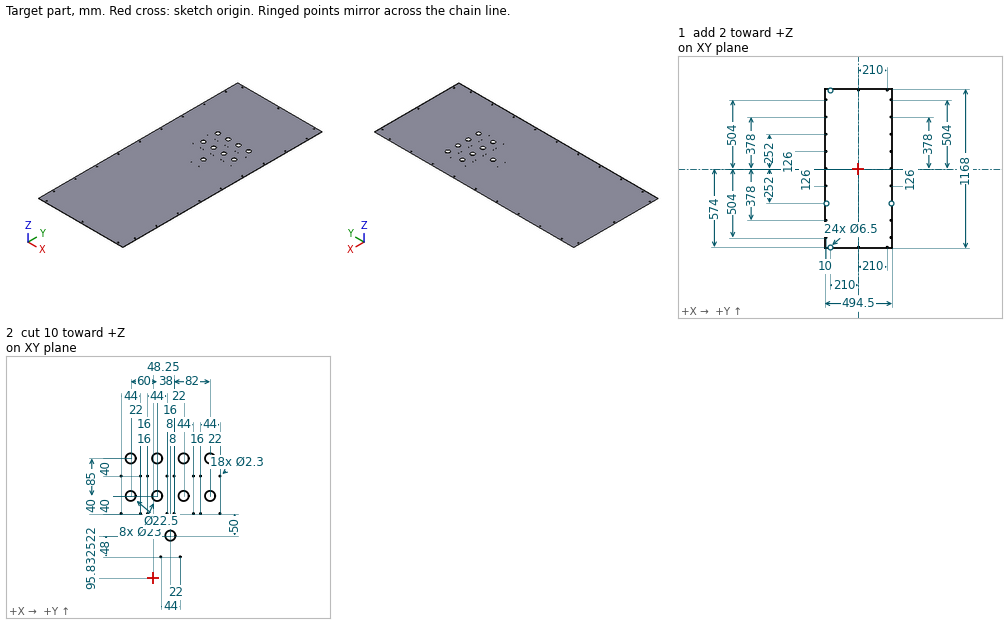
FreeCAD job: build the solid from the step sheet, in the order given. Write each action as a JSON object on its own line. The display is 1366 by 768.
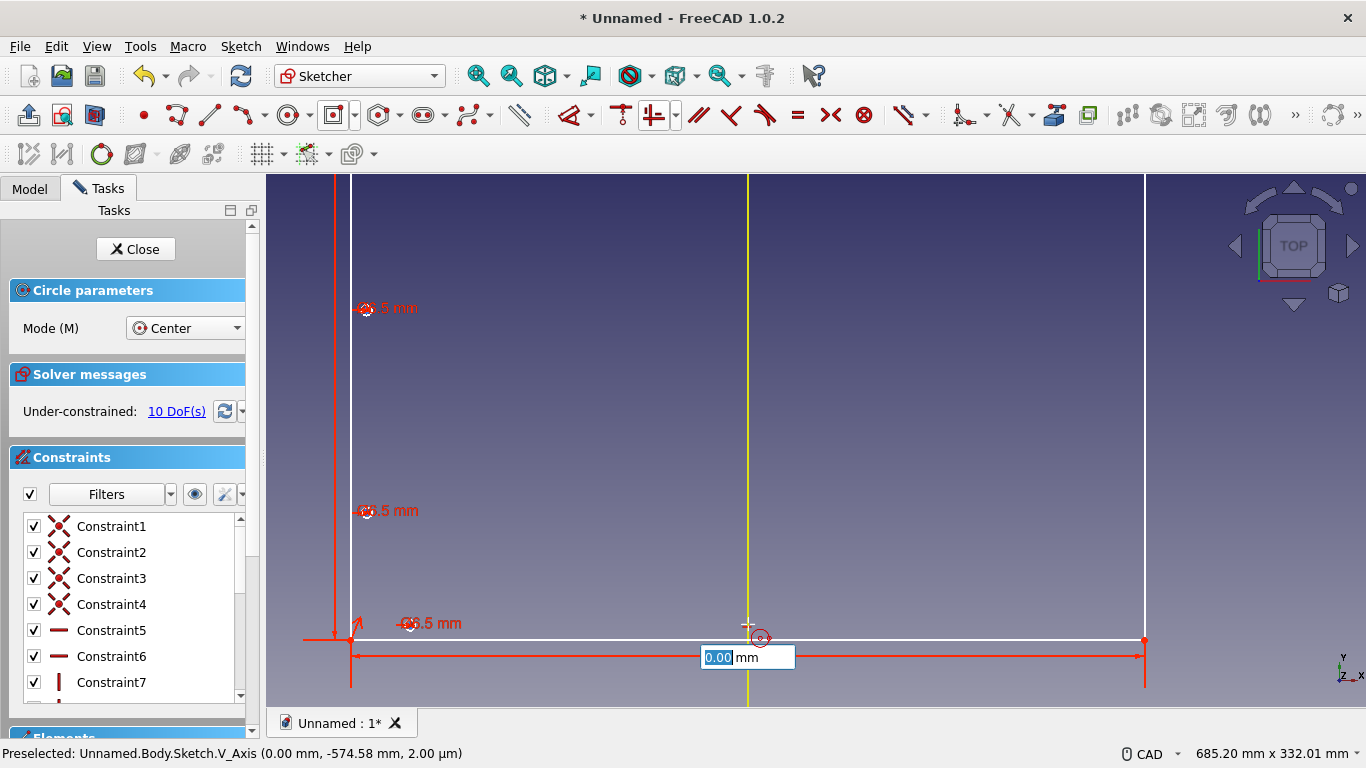
{"action": "scroll", "coordinate": [753, 622], "scroll_direction": "up", "scroll_amount": 6}
{"action": "mouse_move", "coordinate": [750, 621]}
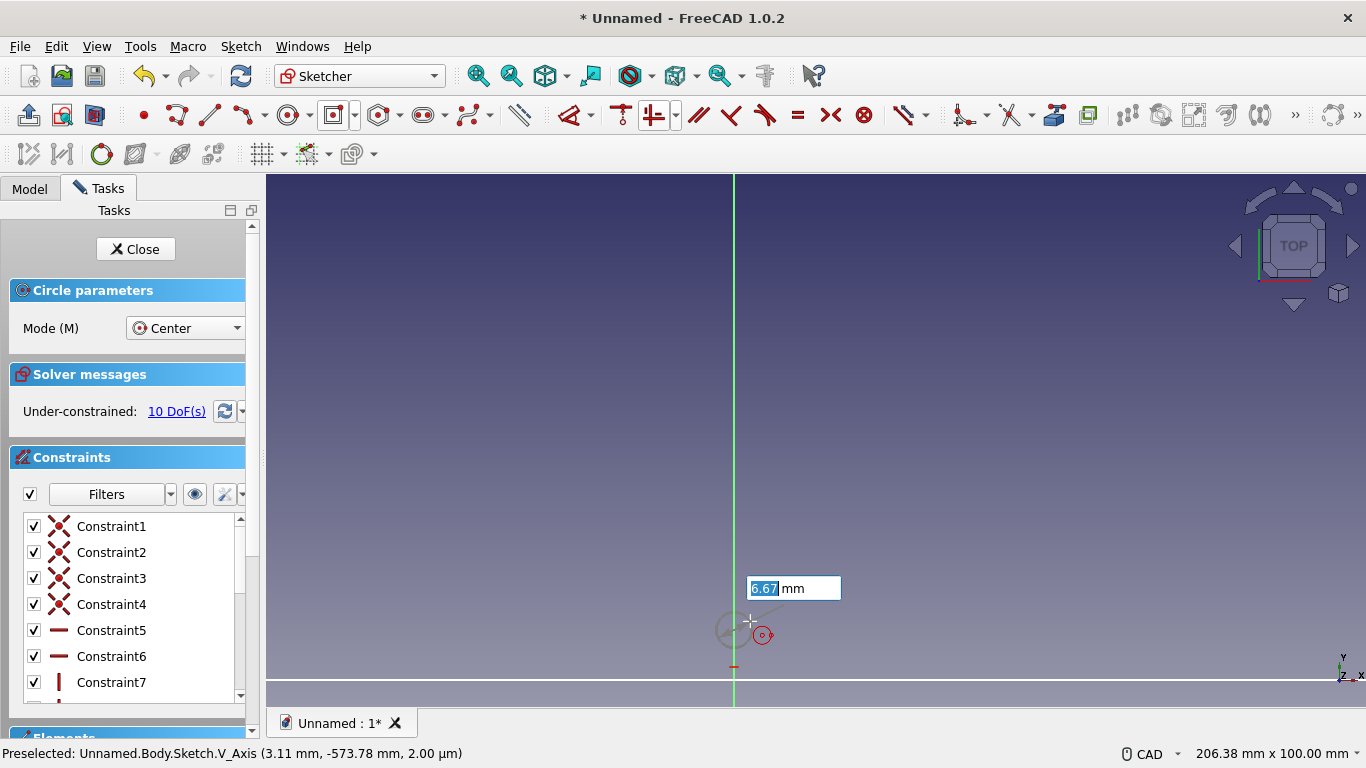
{"action": "type", "text": "6.5"}
{"action": "key", "text": "Return"}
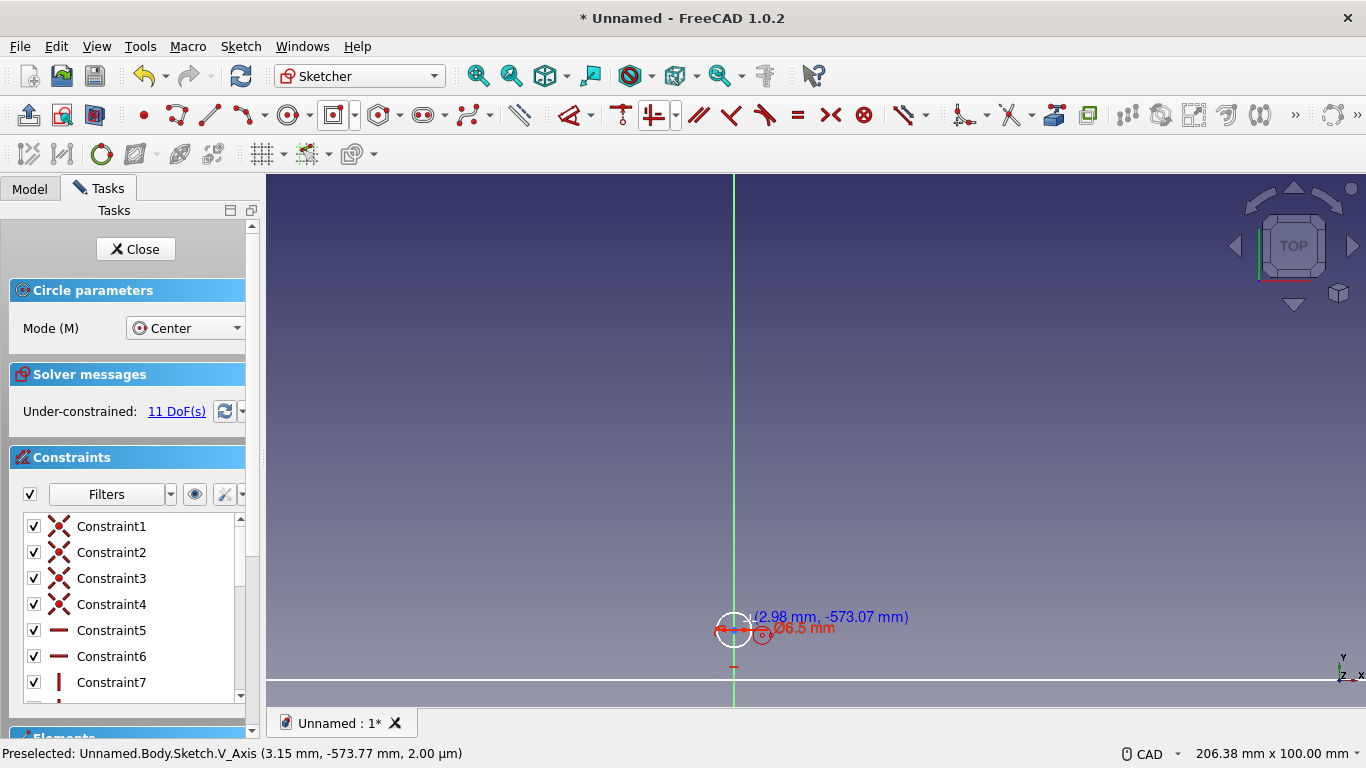
{"action": "scroll", "coordinate": [748, 591], "scroll_direction": "down", "scroll_amount": 15}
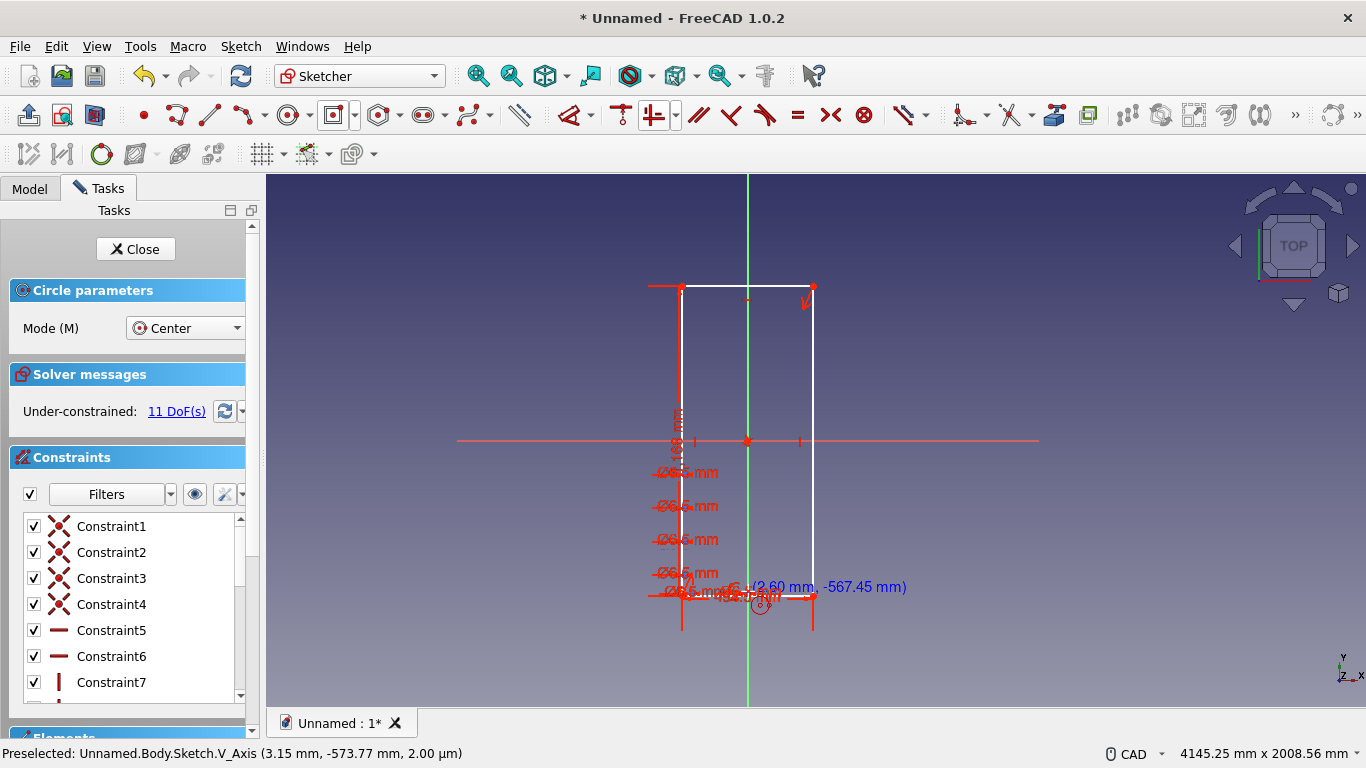
{"action": "scroll", "coordinate": [803, 594], "scroll_direction": "up", "scroll_amount": 17}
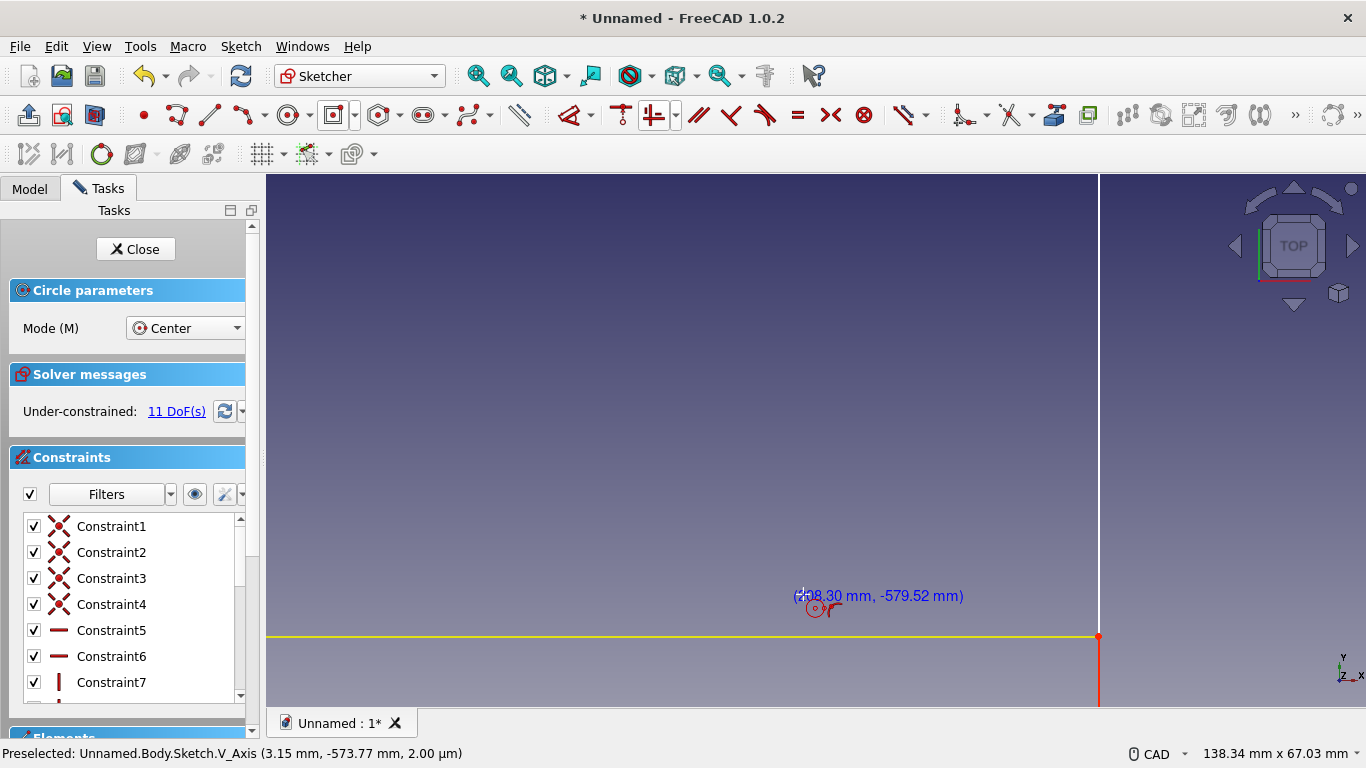
{"action": "scroll", "coordinate": [816, 629], "scroll_direction": "down", "scroll_amount": 16}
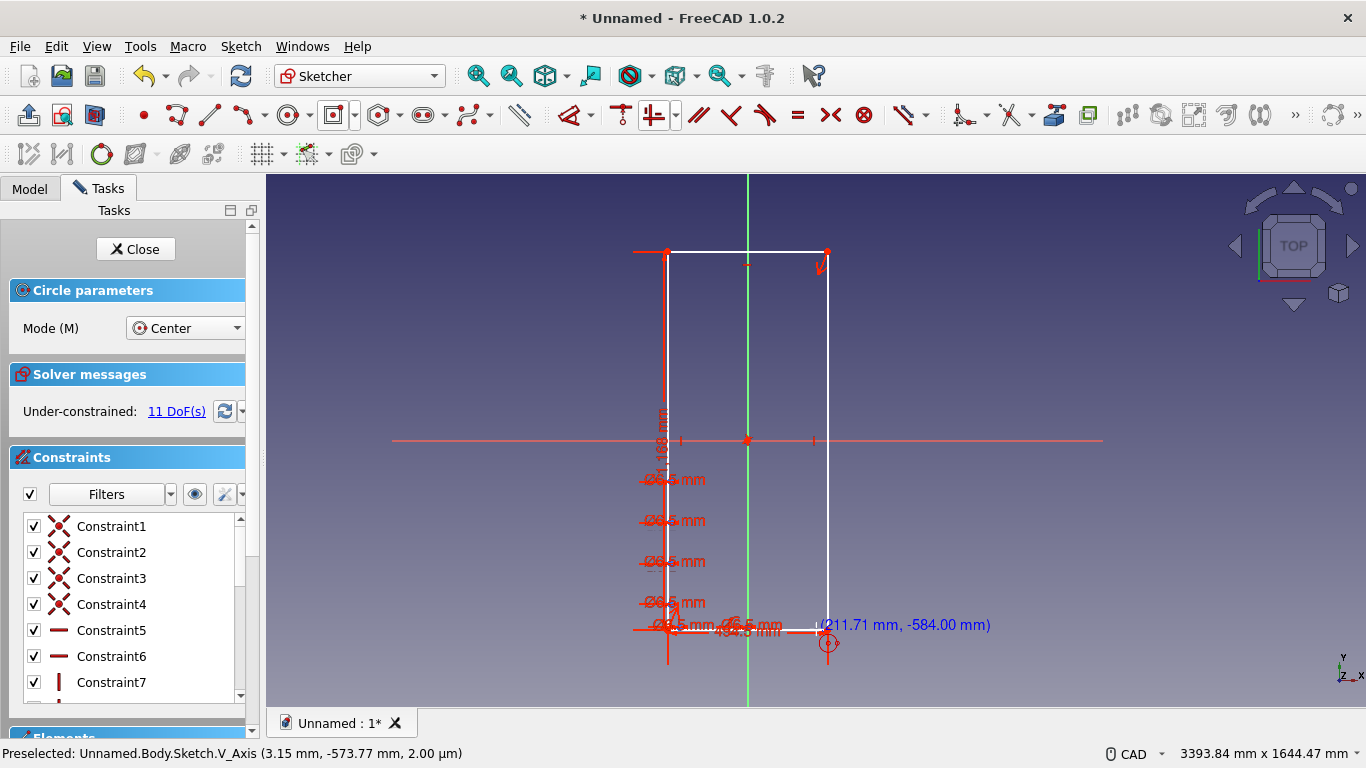
{"action": "scroll", "coordinate": [816, 627], "scroll_direction": "up", "scroll_amount": 8}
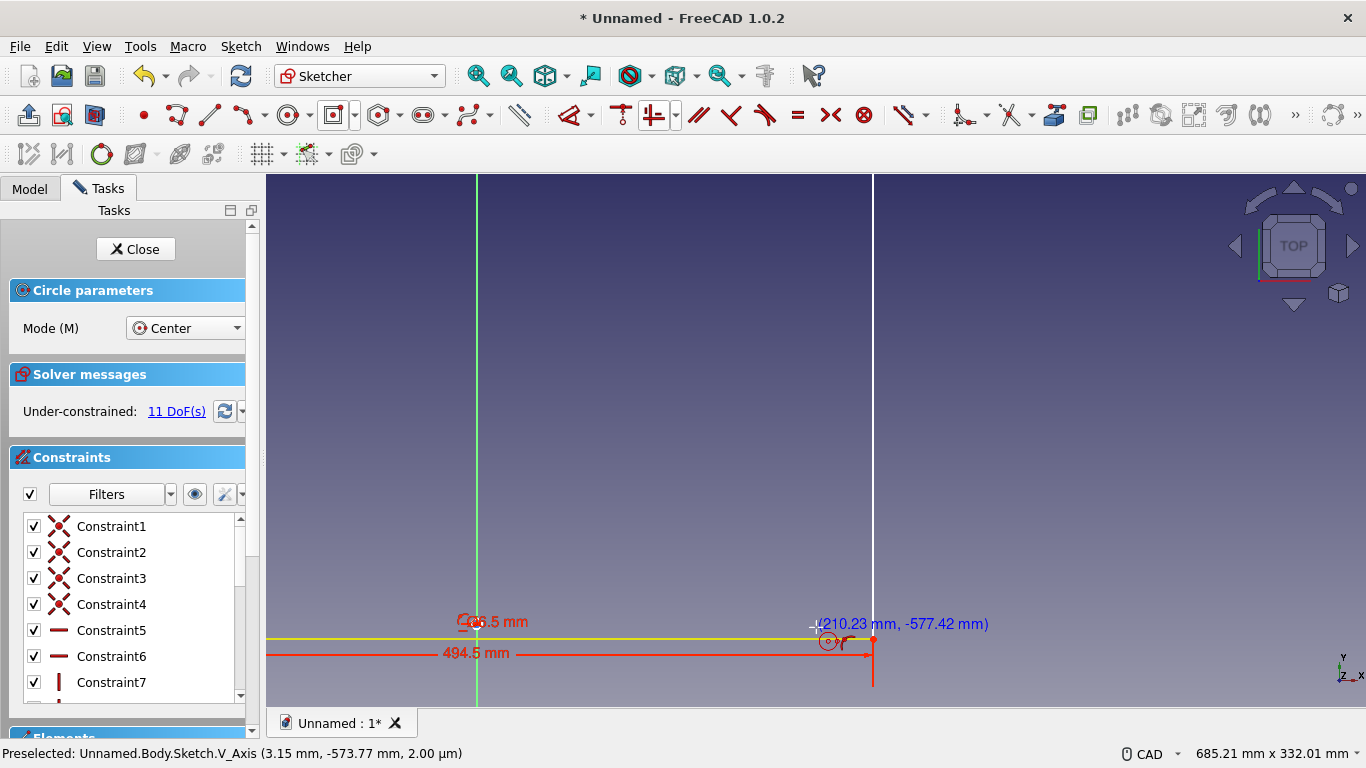
{"action": "left_click", "coordinate": [814, 623]}
{"action": "mouse_move", "coordinate": [817, 619]}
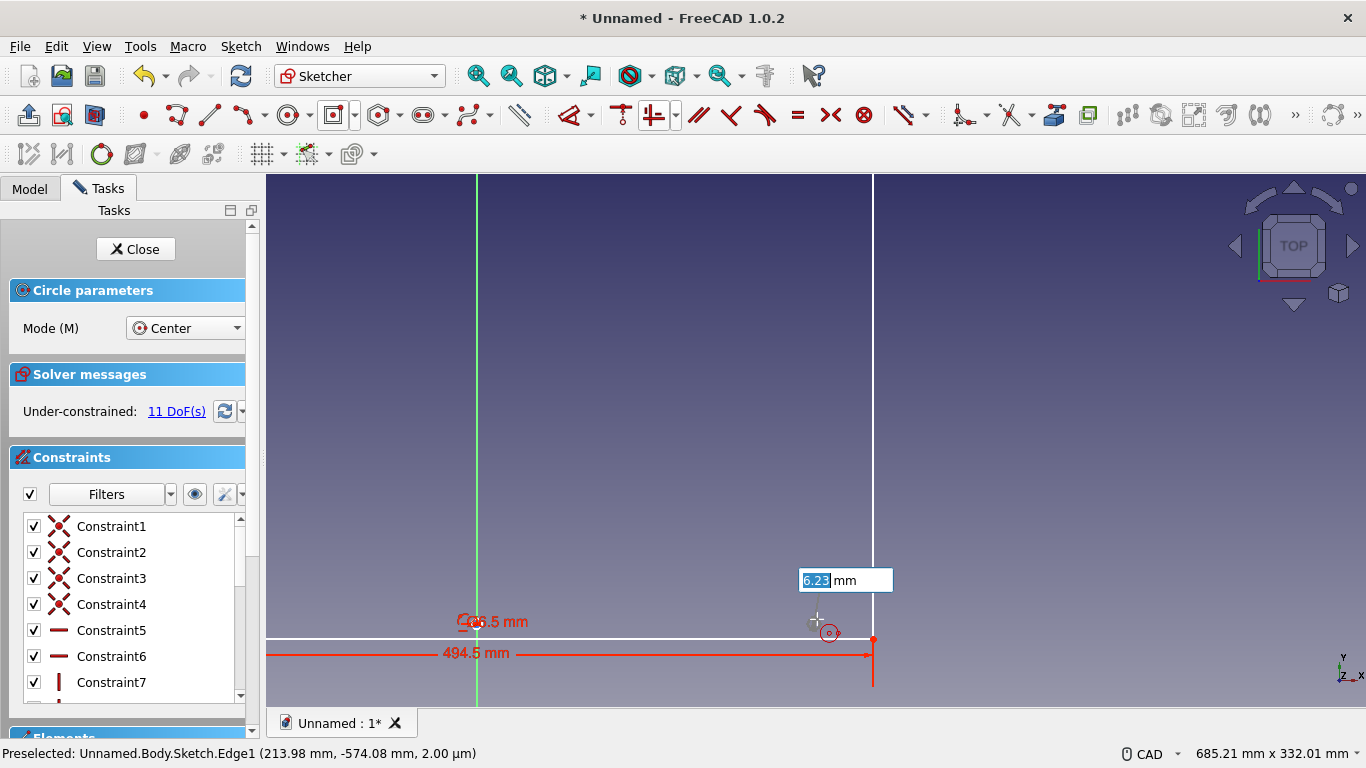
{"action": "type", "text": "6.5"}
{"action": "key", "text": "Return"}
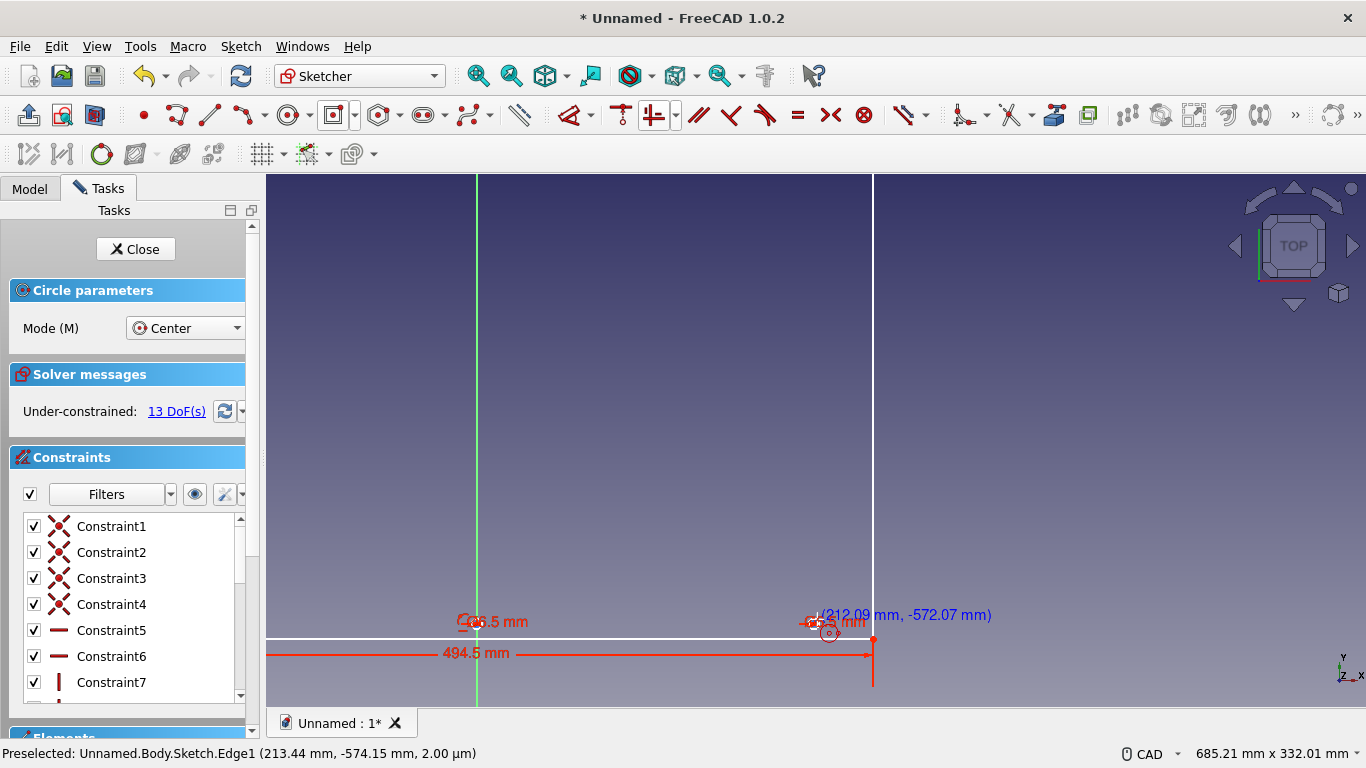
{"action": "scroll", "coordinate": [857, 511], "scroll_direction": "up", "scroll_amount": 8}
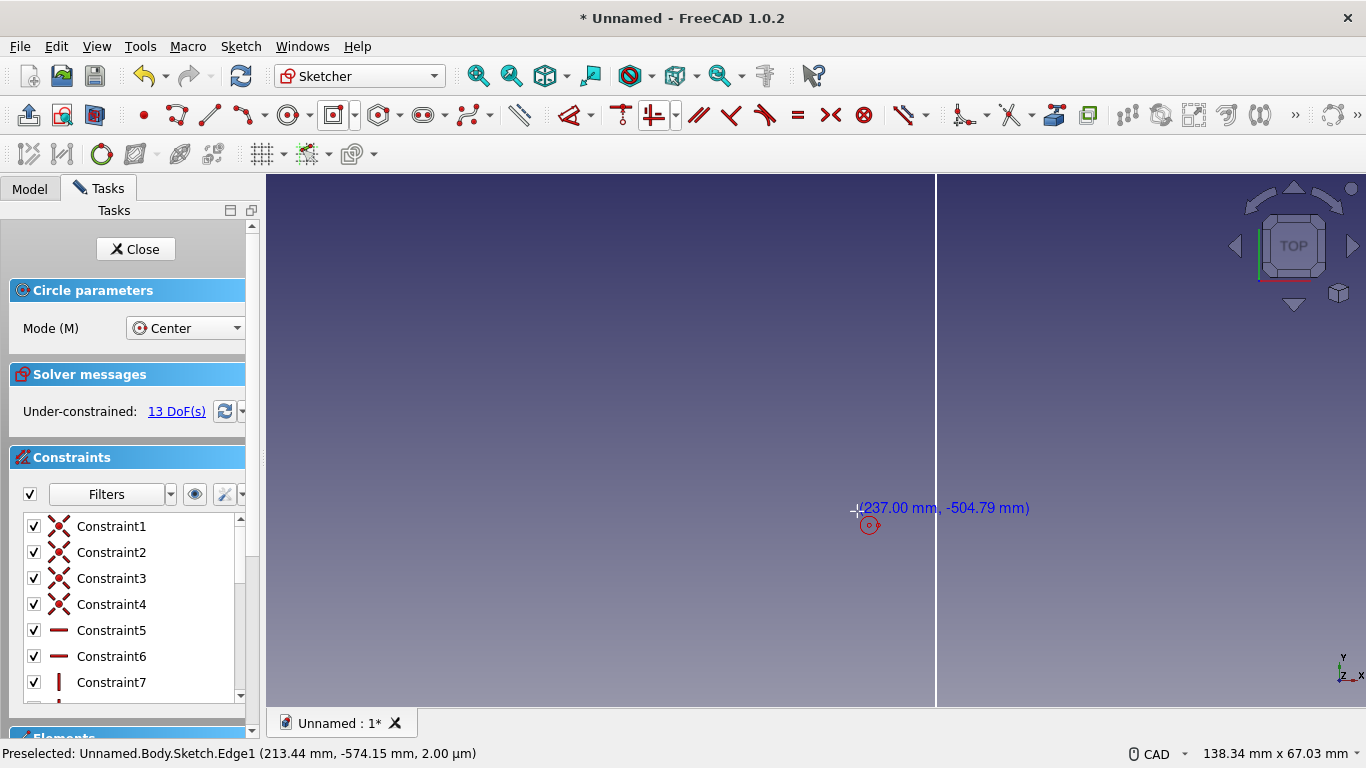
{"action": "scroll", "coordinate": [823, 608], "scroll_direction": "down", "scroll_amount": 16}